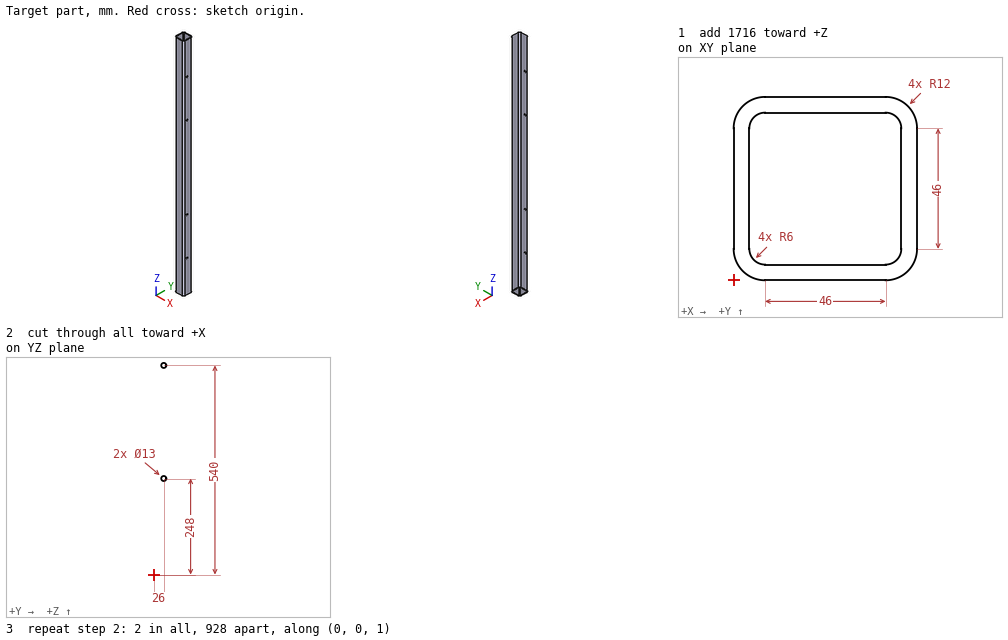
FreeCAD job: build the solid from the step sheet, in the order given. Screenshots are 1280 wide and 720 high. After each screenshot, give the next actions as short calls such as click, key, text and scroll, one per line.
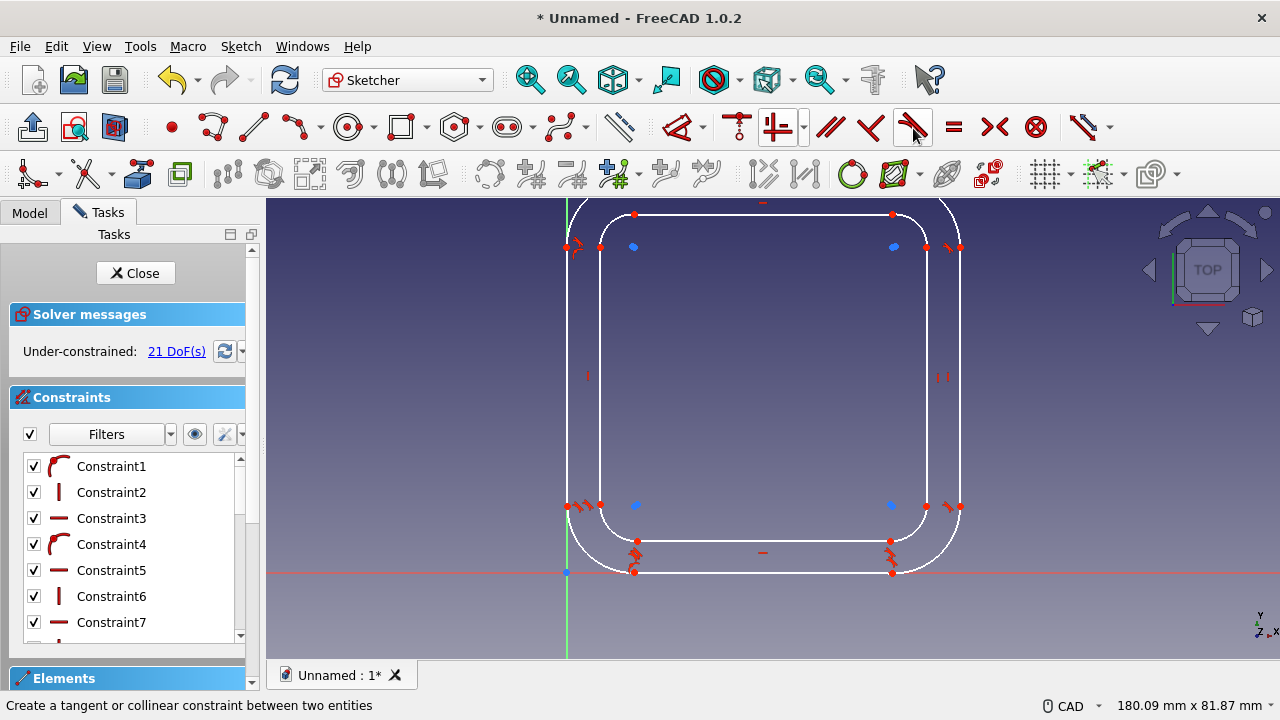
click(600, 427)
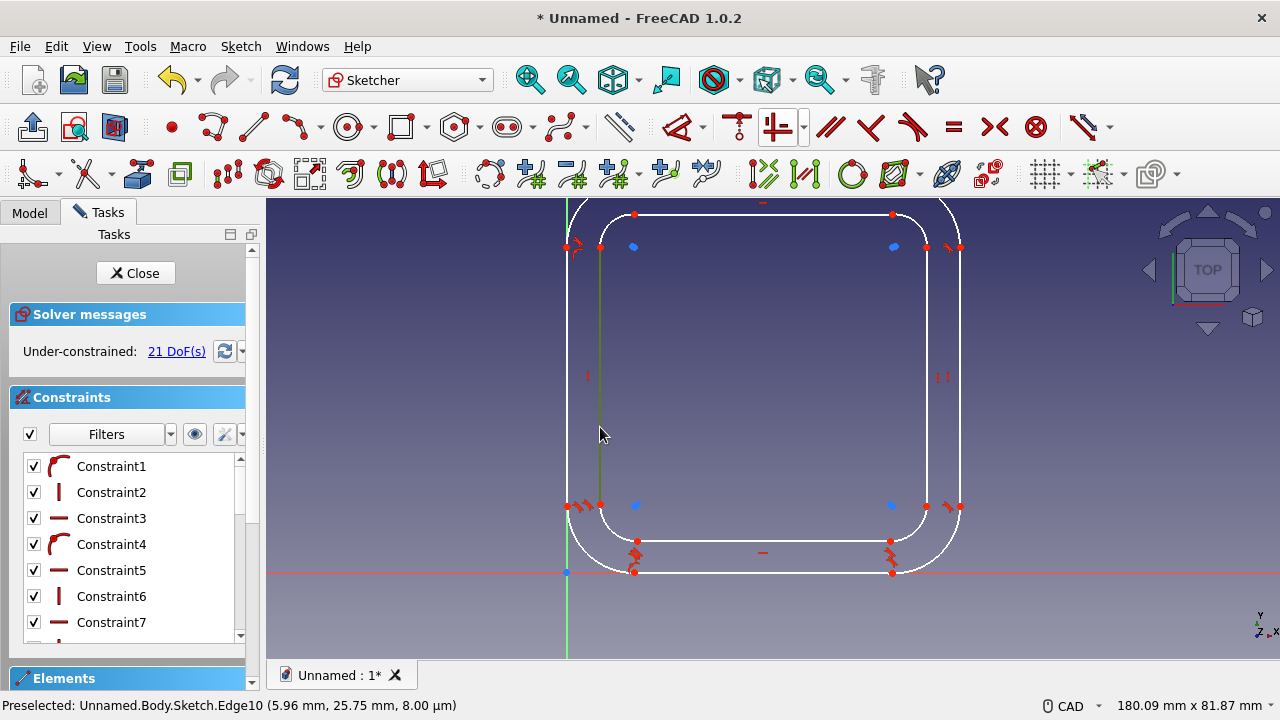
click(604, 232)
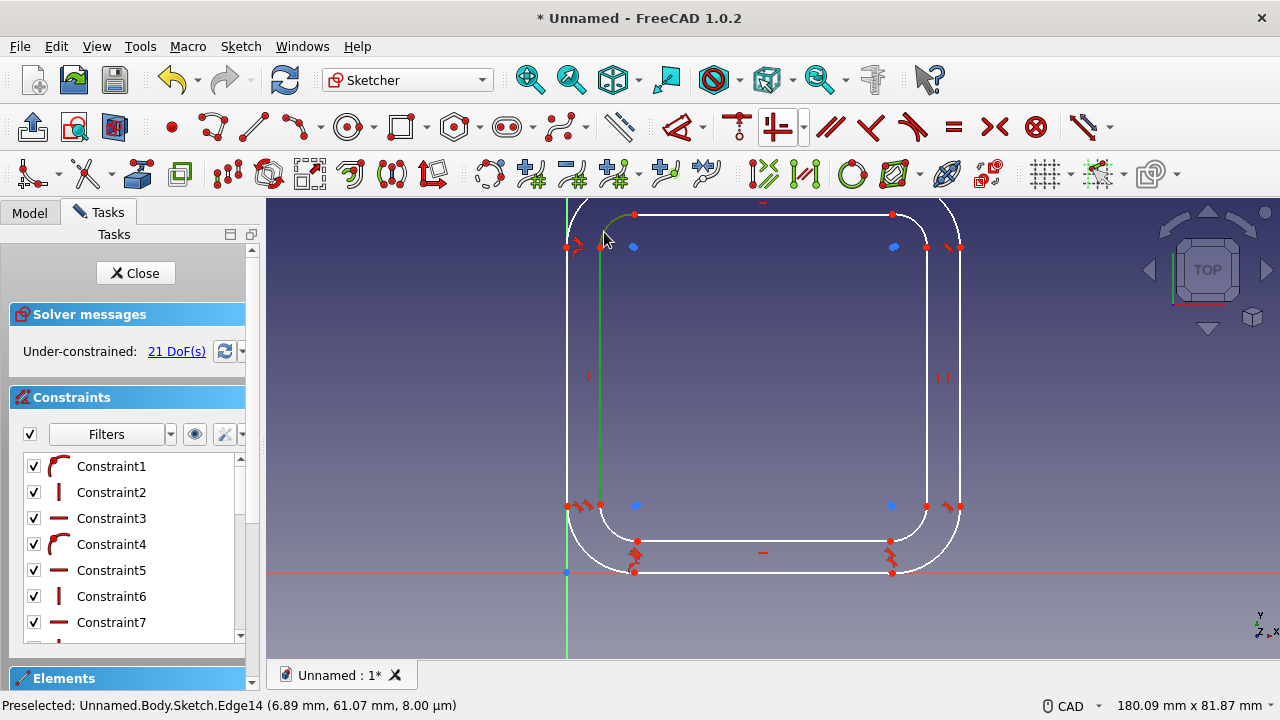
click(913, 128)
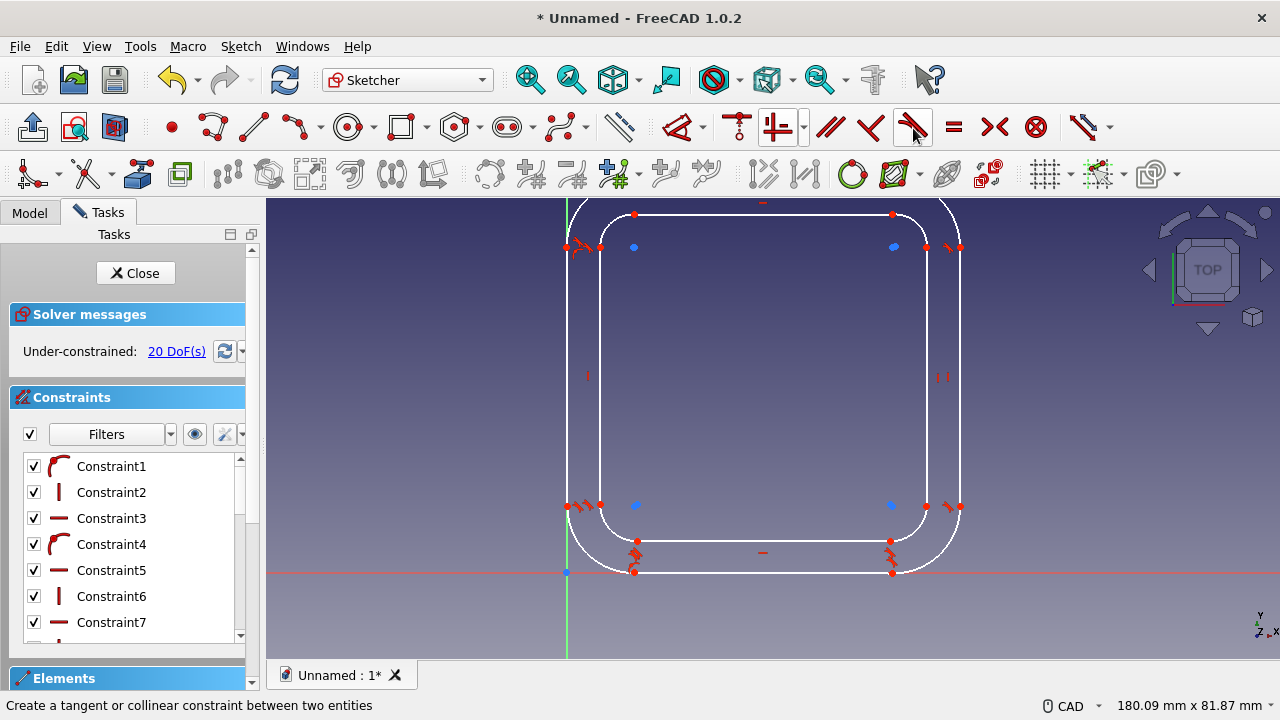
scroll(584, 535, down, 2)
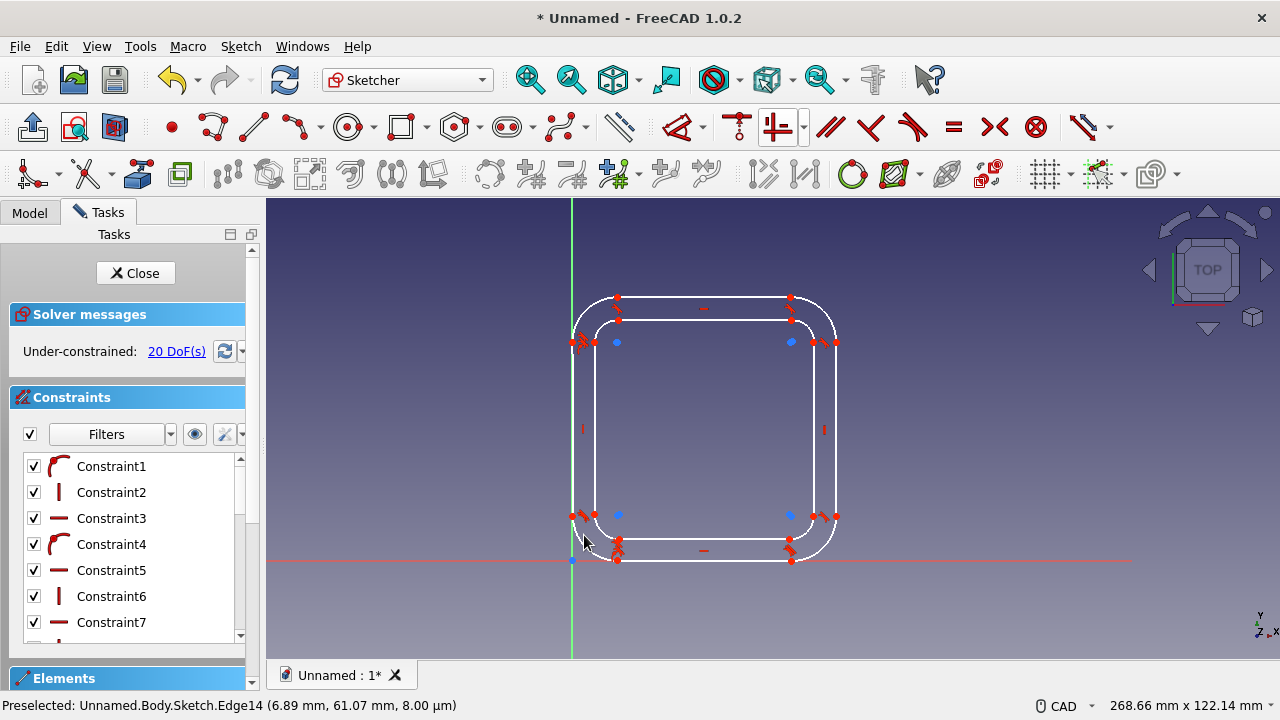
click(670, 320)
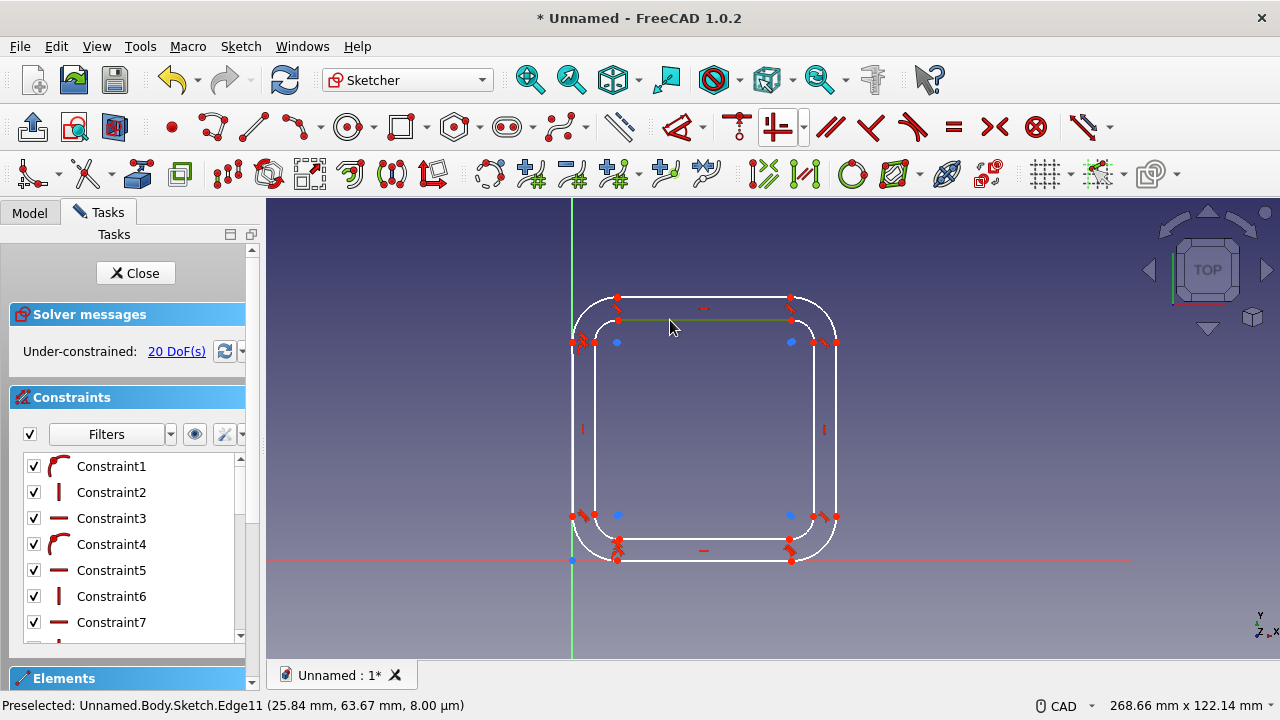
scroll(608, 322, up, 2)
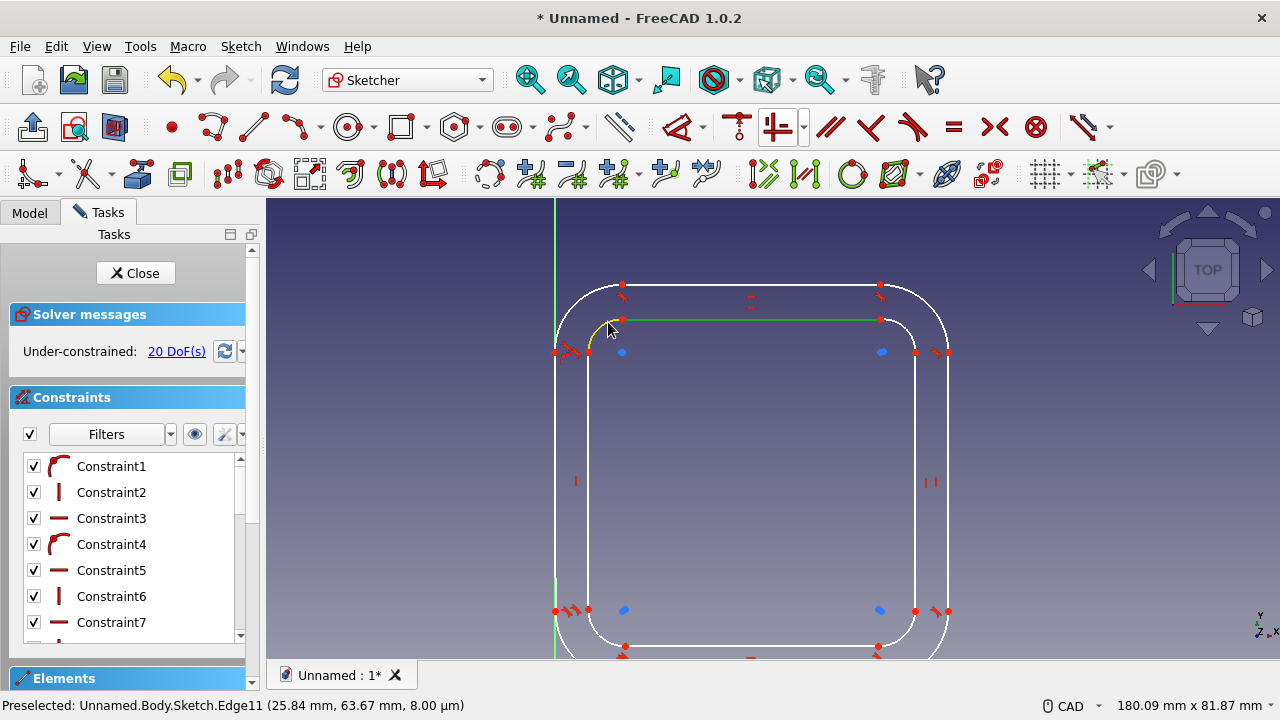
click(607, 323)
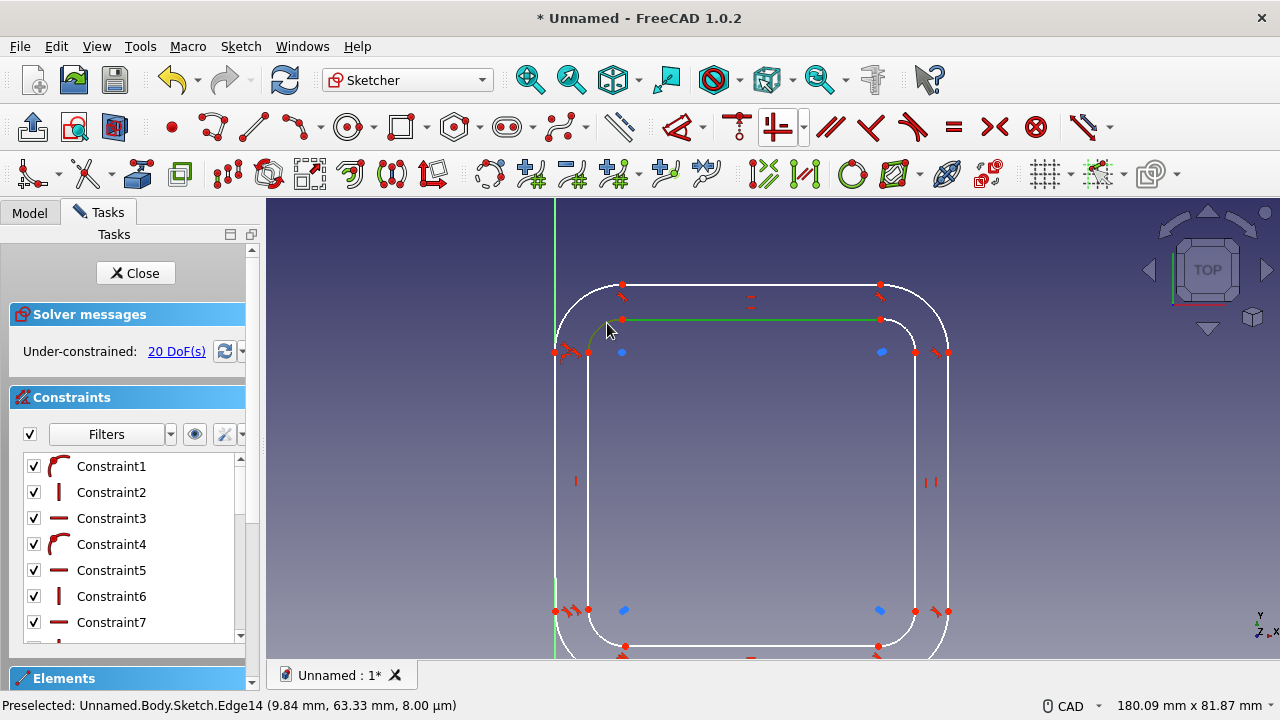
click(913, 128)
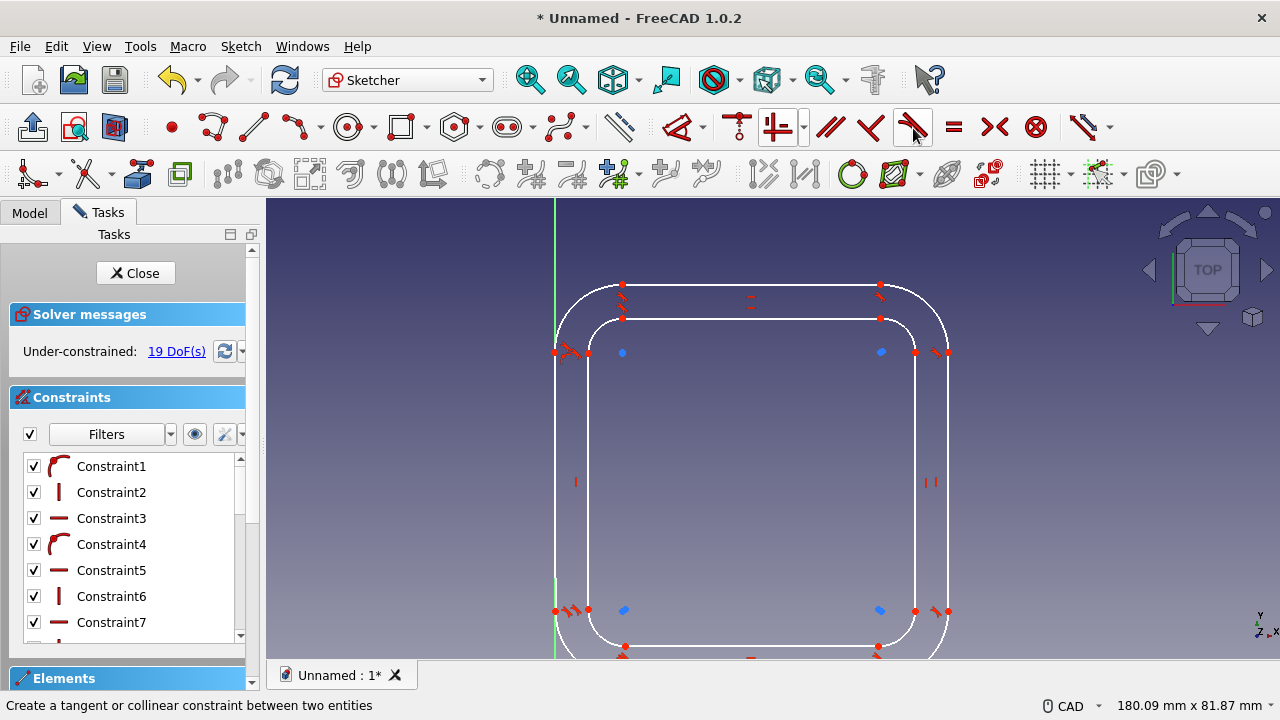
click(700, 319)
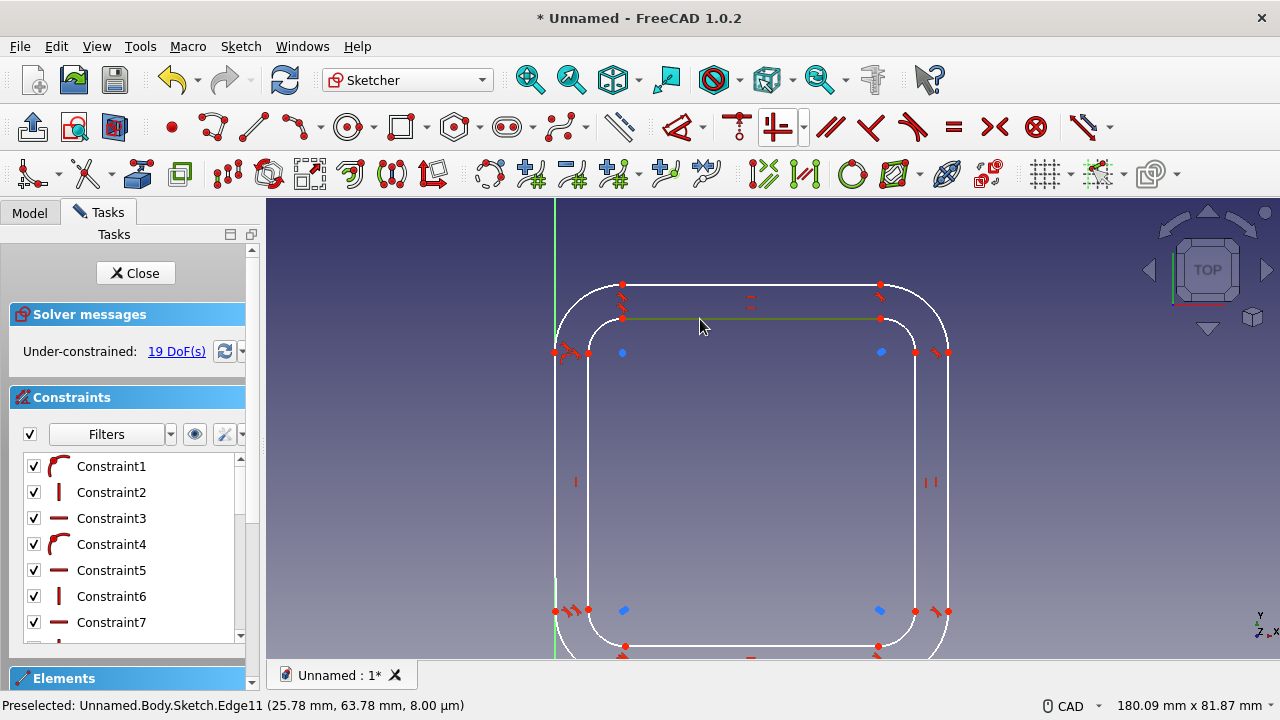
click(912, 337)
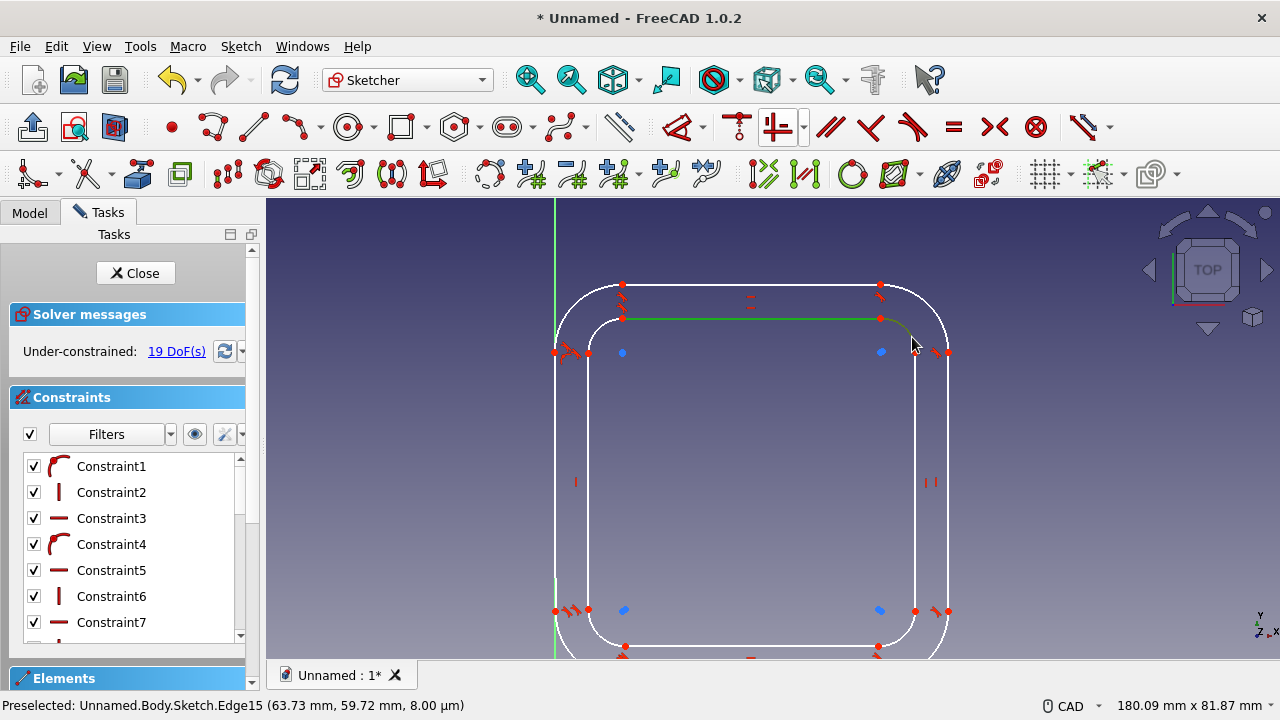
click(913, 128)